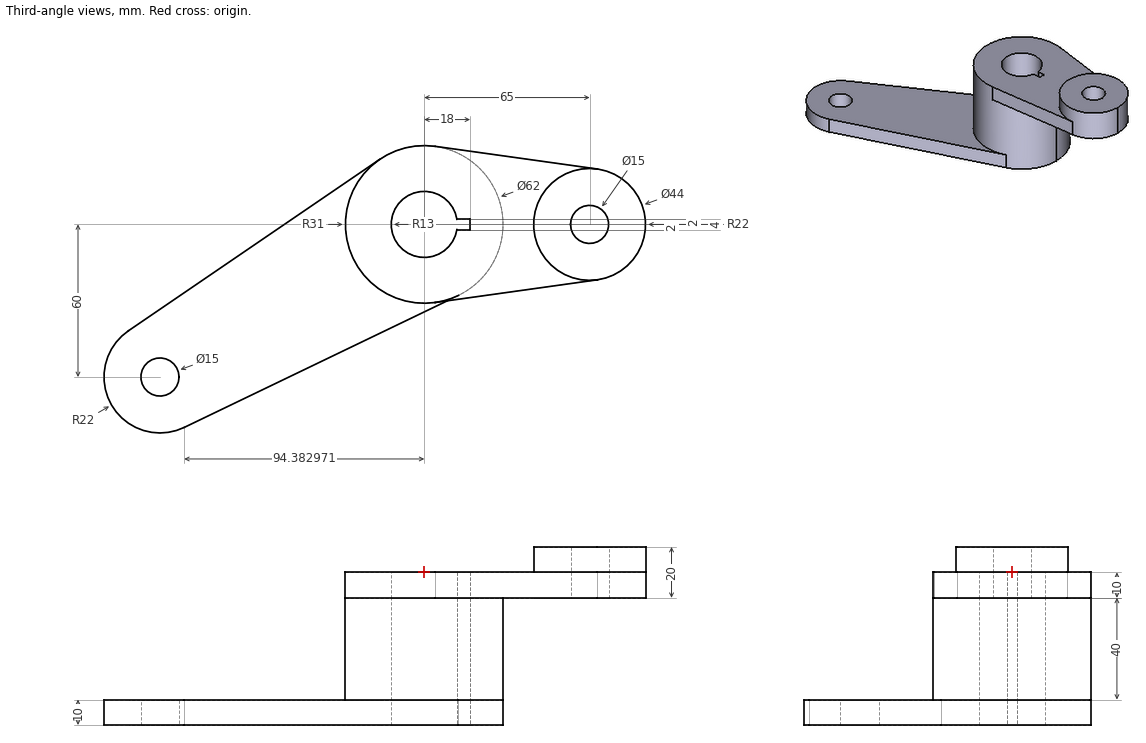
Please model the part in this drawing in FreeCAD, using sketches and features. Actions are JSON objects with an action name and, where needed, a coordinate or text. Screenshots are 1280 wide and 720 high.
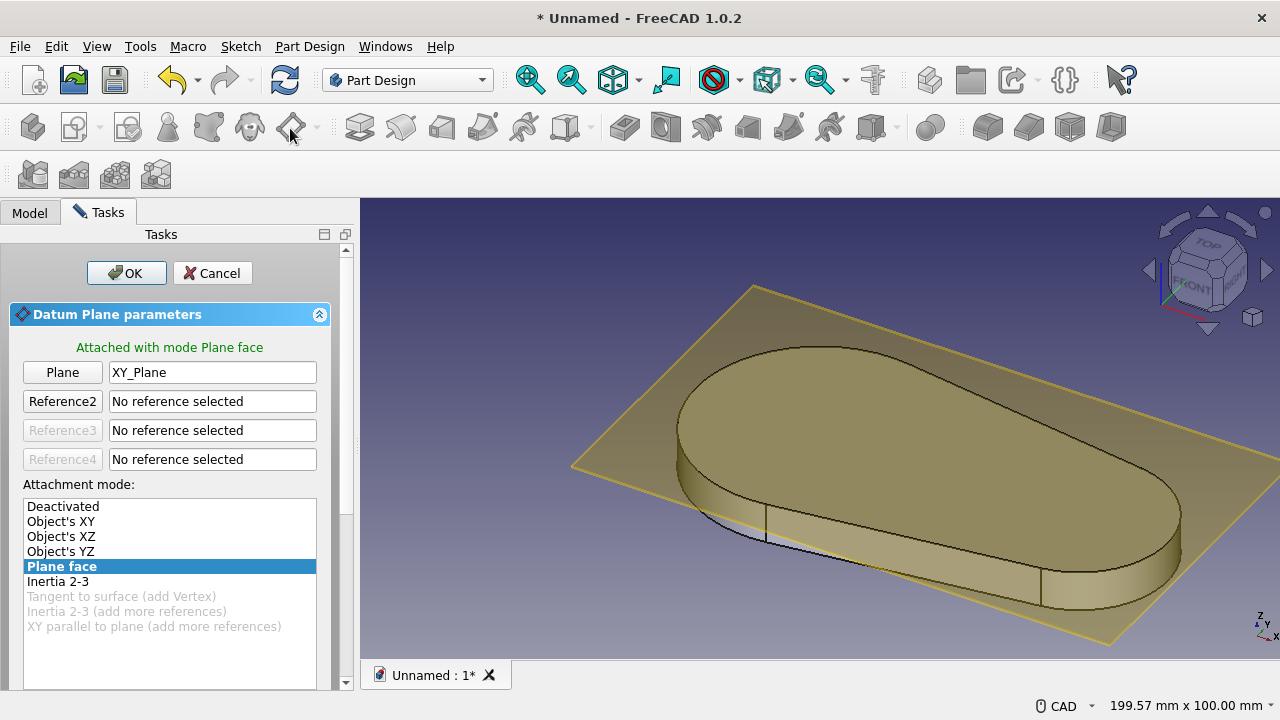
{"action": "scroll", "coordinate": [346, 467], "scroll_direction": "down", "scroll_amount": 4}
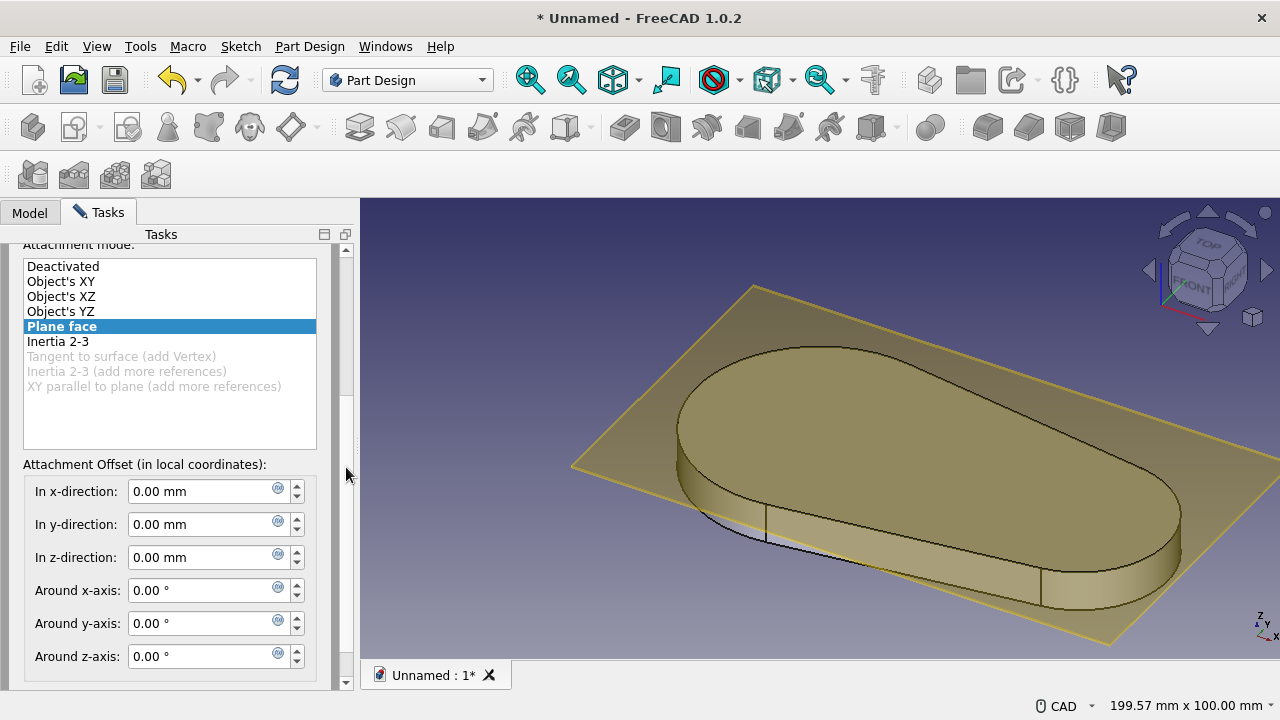
{"action": "triple_click", "coordinate": [210, 558]}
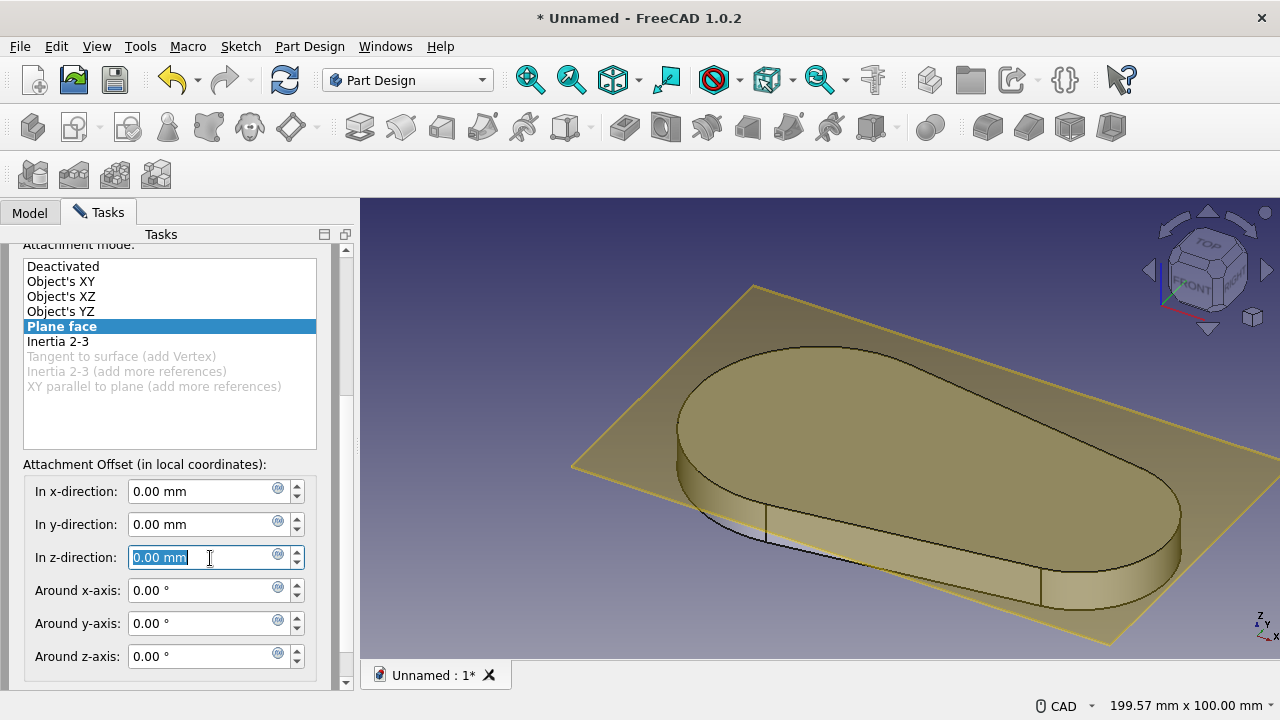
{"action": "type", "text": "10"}
{"action": "key", "text": "Tab"}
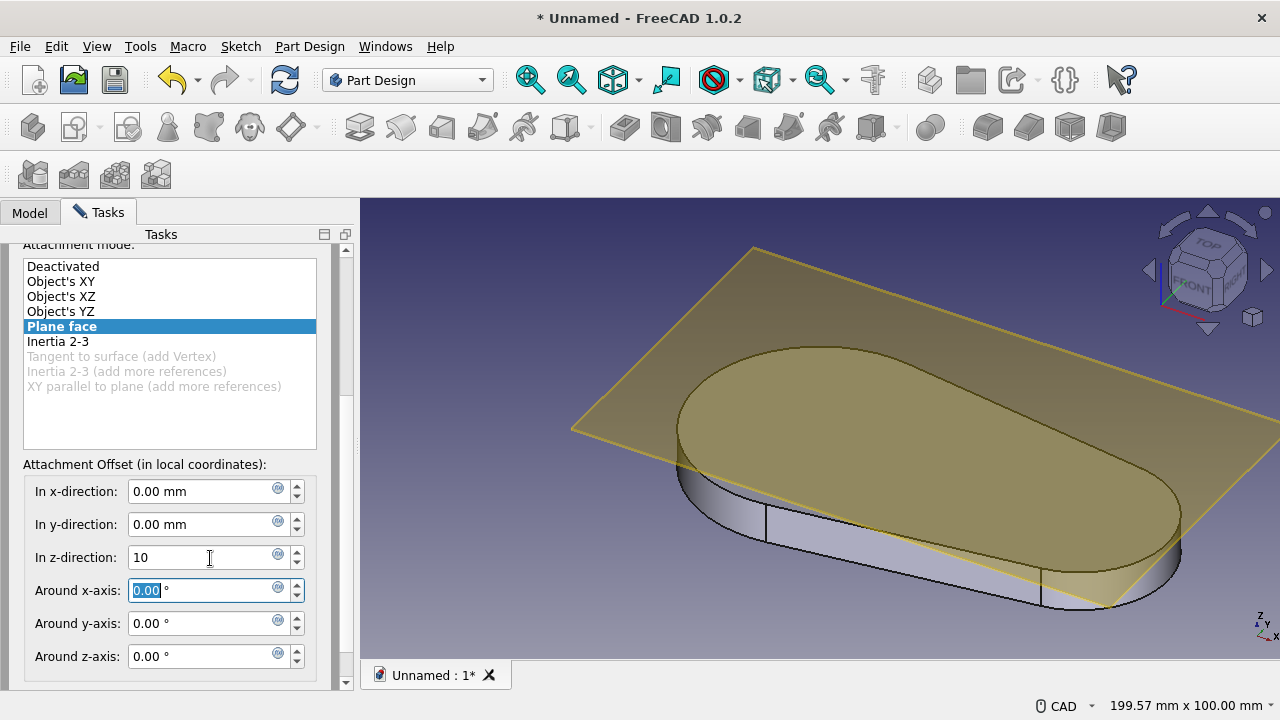
{"action": "scroll", "coordinate": [346, 467], "scroll_direction": "up", "scroll_amount": 5}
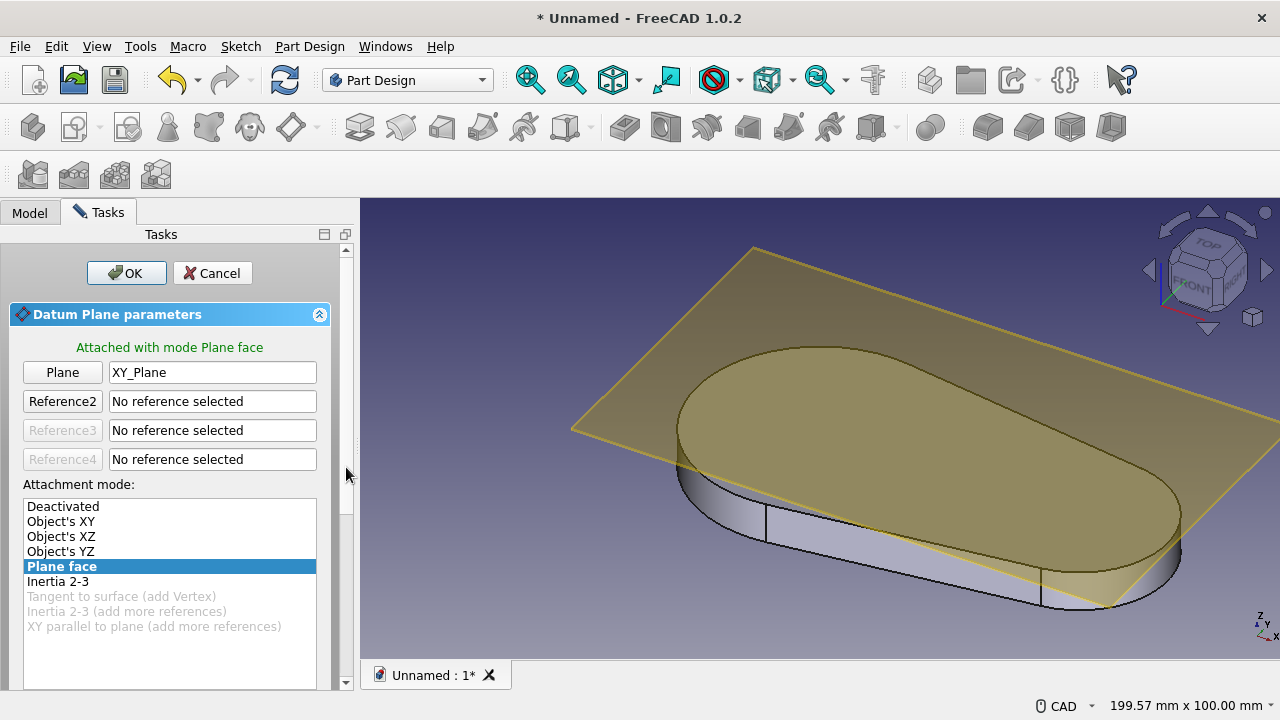
{"action": "left_click", "coordinate": [127, 273]}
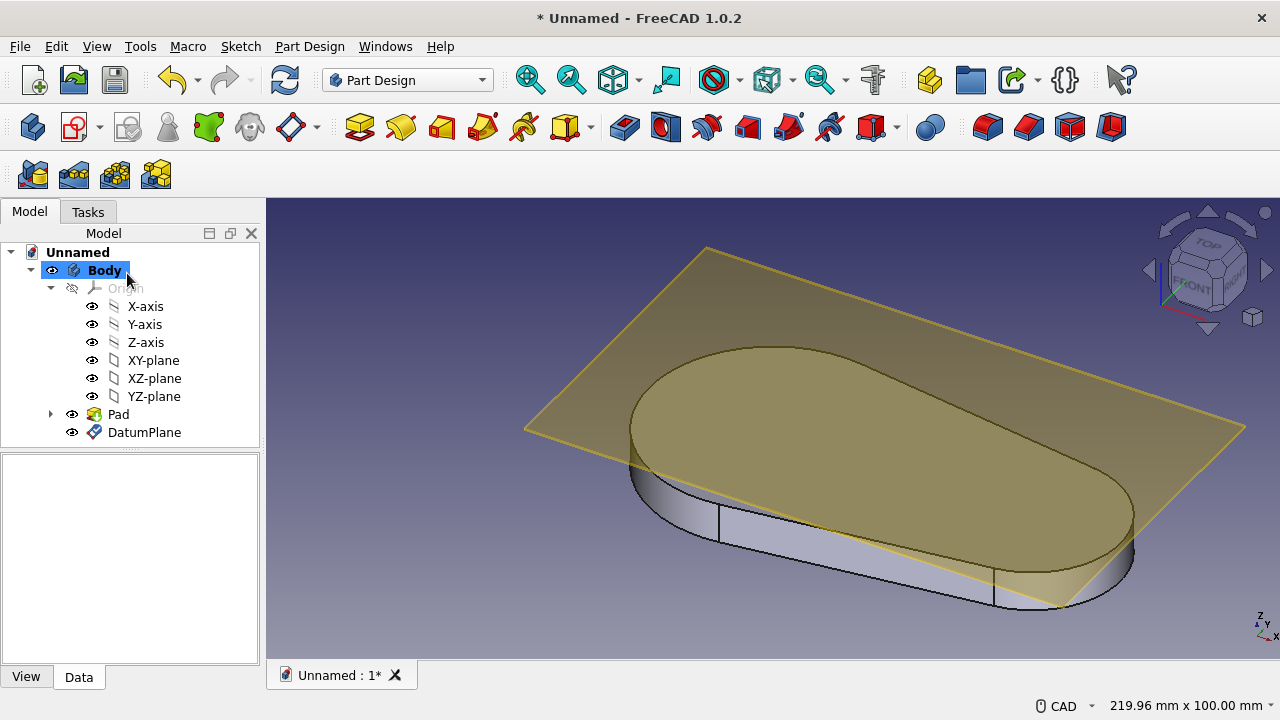
{"action": "left_click", "coordinate": [117, 432]}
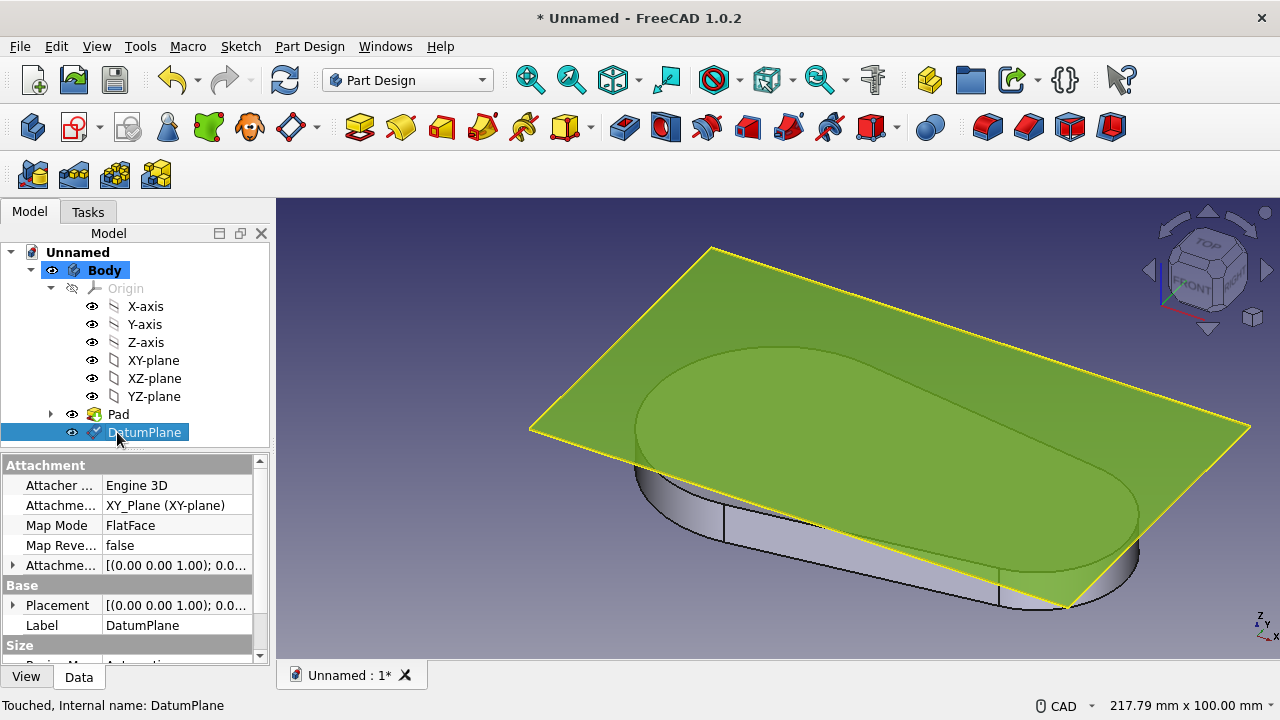
{"action": "left_click", "coordinate": [74, 128]}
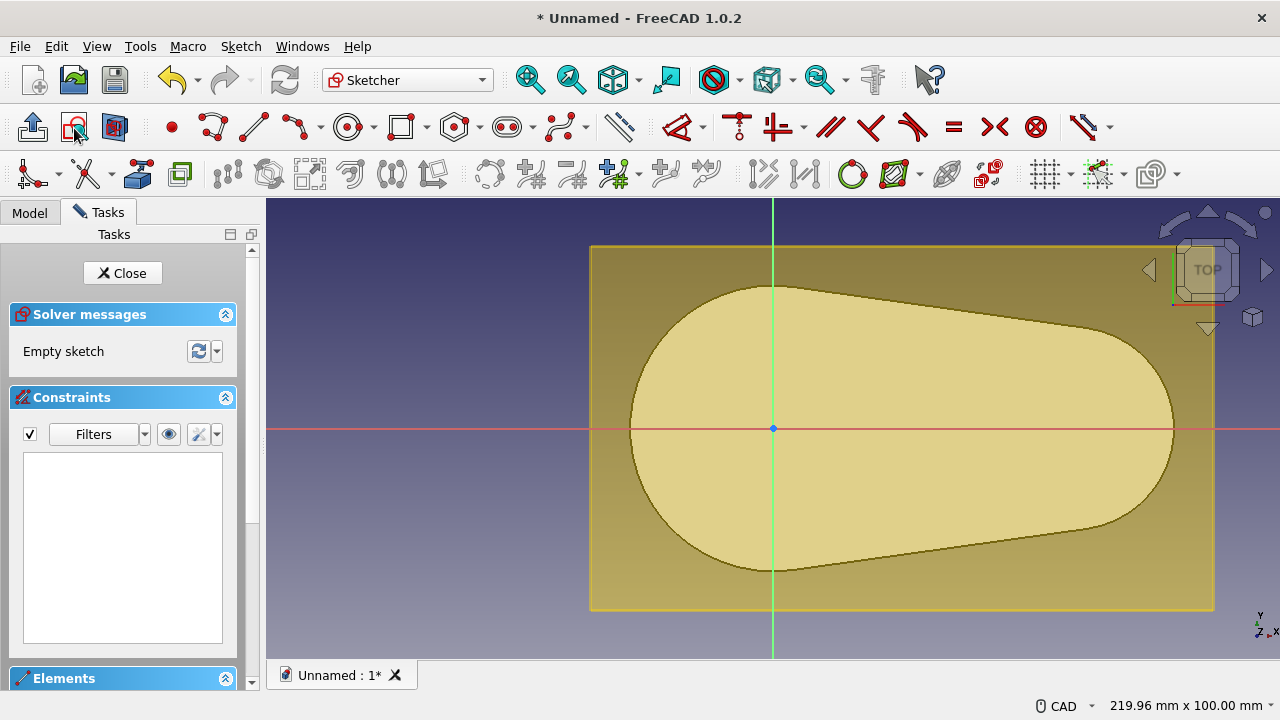
{"action": "scroll", "coordinate": [294, 428], "scroll_direction": "down", "scroll_amount": 1}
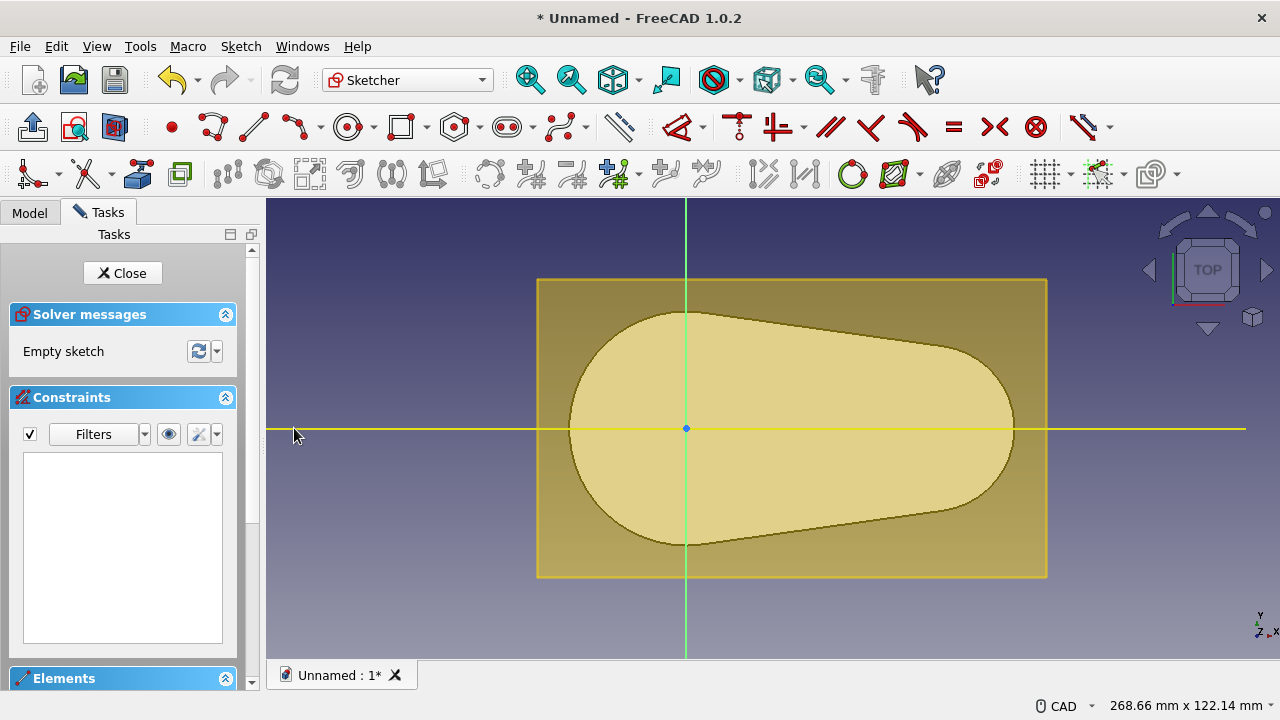
{"action": "scroll", "coordinate": [1028, 428], "scroll_direction": "up", "scroll_amount": 3}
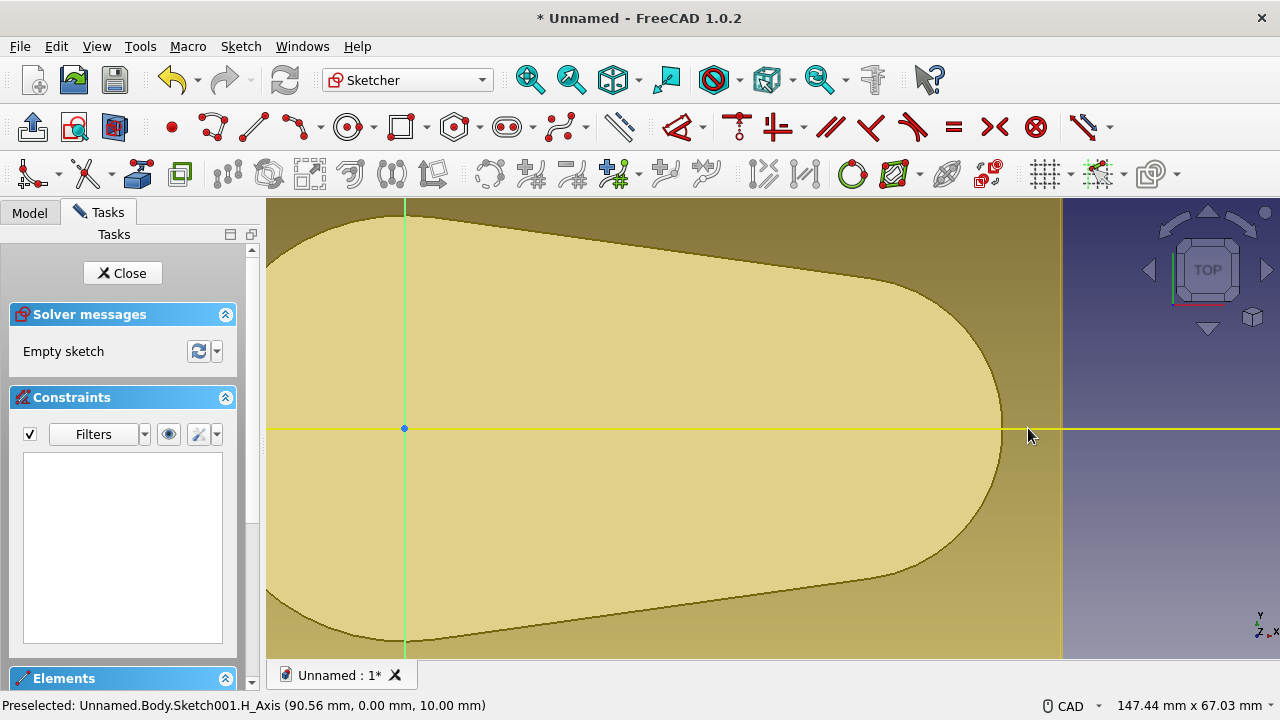
{"action": "key", "text": "g c"}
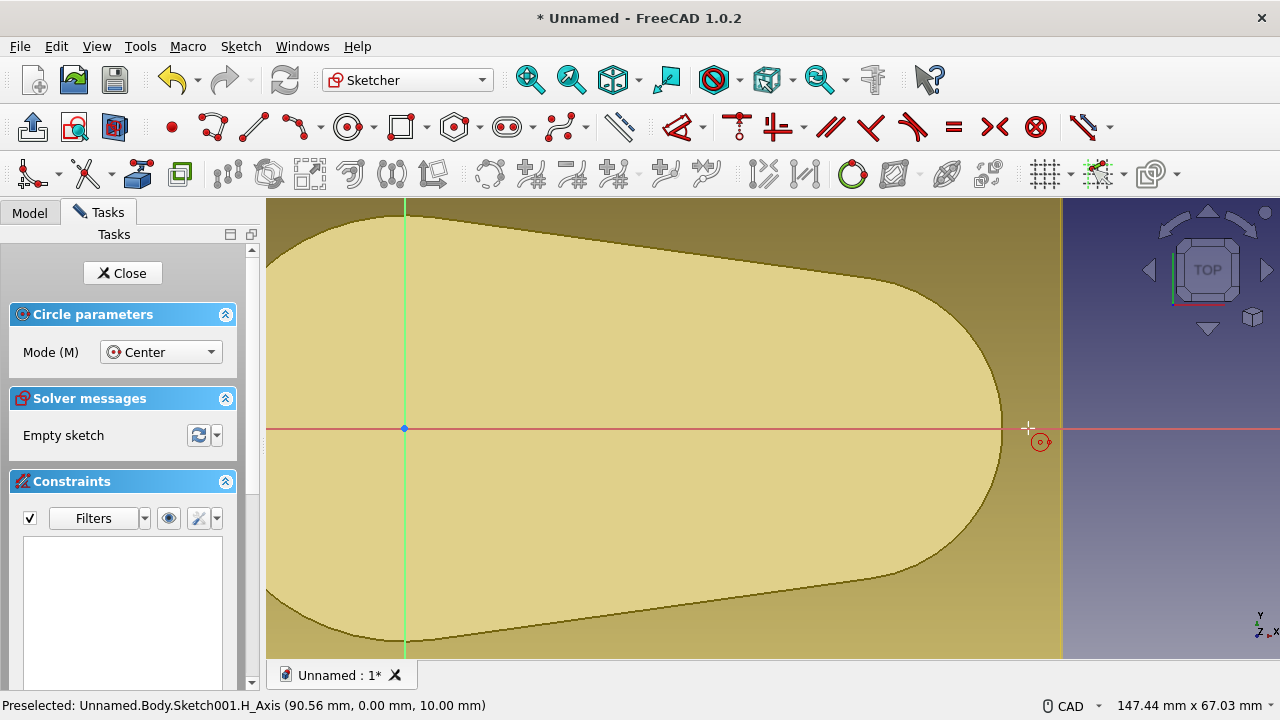
{"action": "left_click", "coordinate": [852, 428]}
{"action": "left_click", "coordinate": [959, 322]}